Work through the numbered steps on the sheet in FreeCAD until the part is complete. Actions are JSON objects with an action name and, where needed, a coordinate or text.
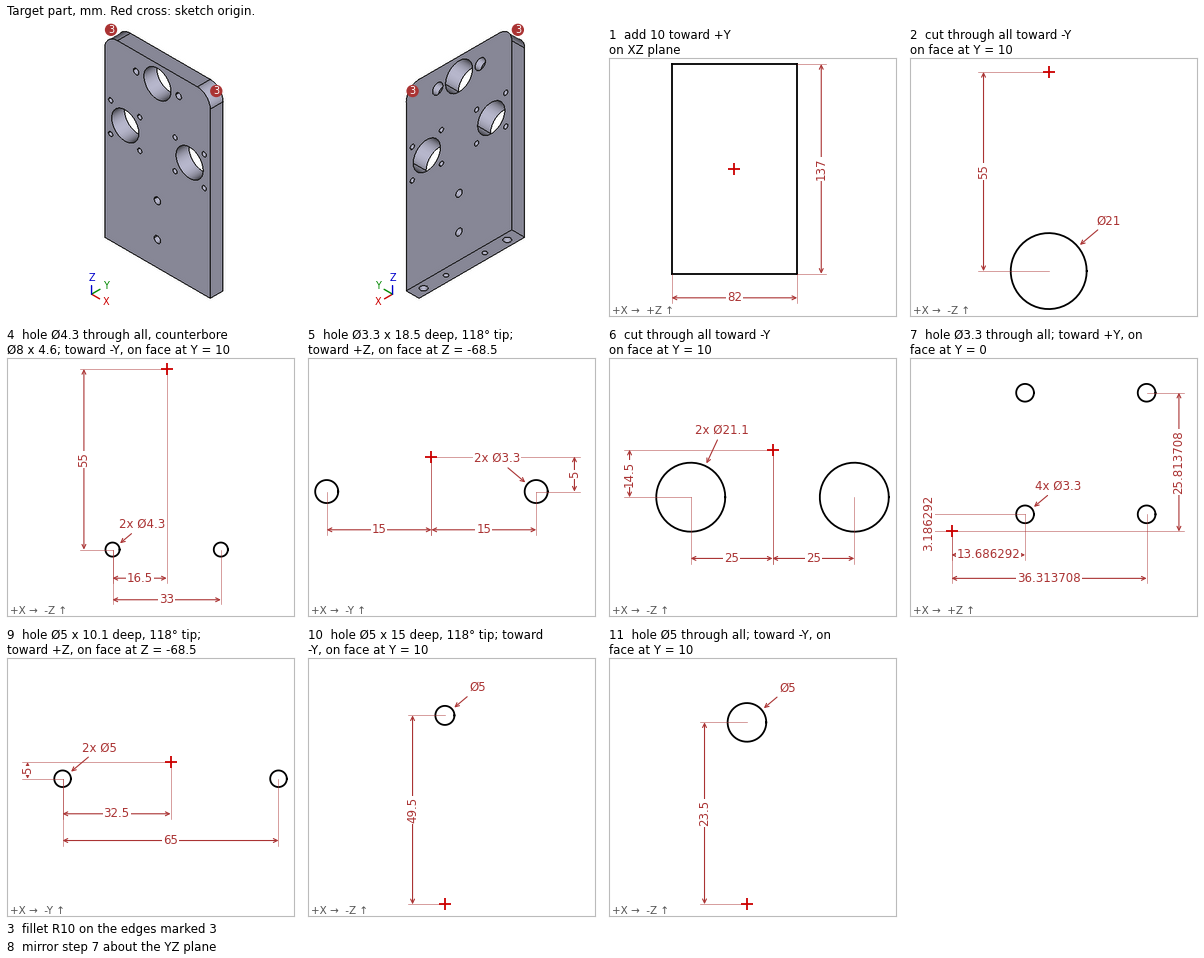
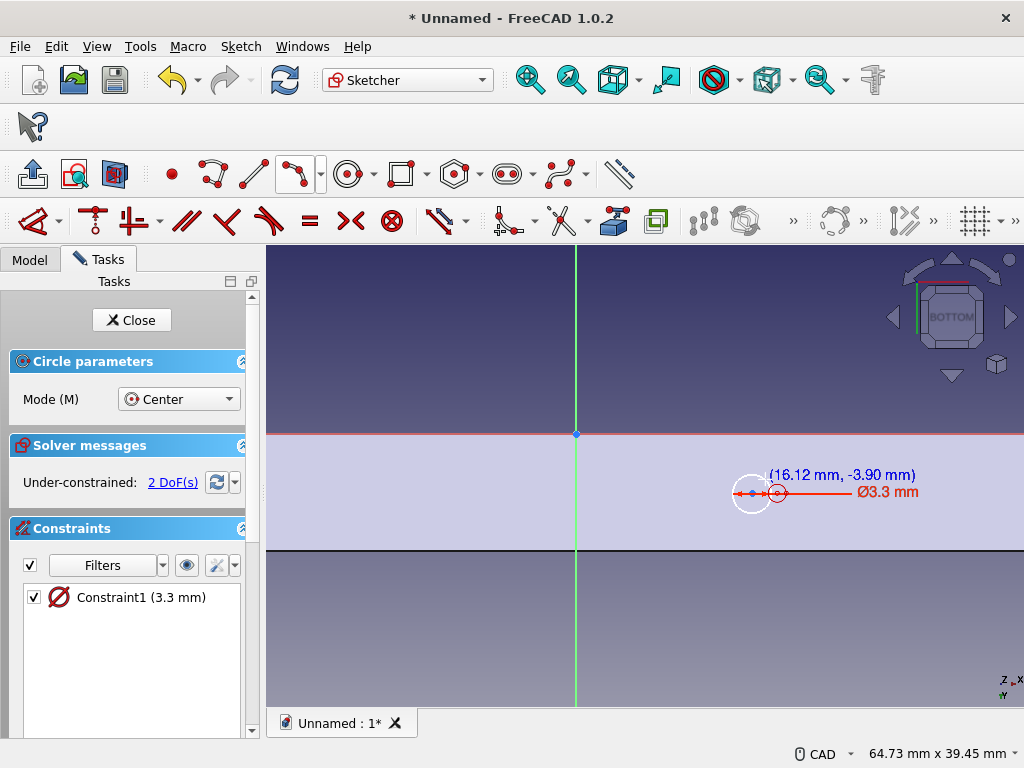
{"action": "left_click", "coordinate": [401, 493]}
{"action": "mouse_move", "coordinate": [414, 479]}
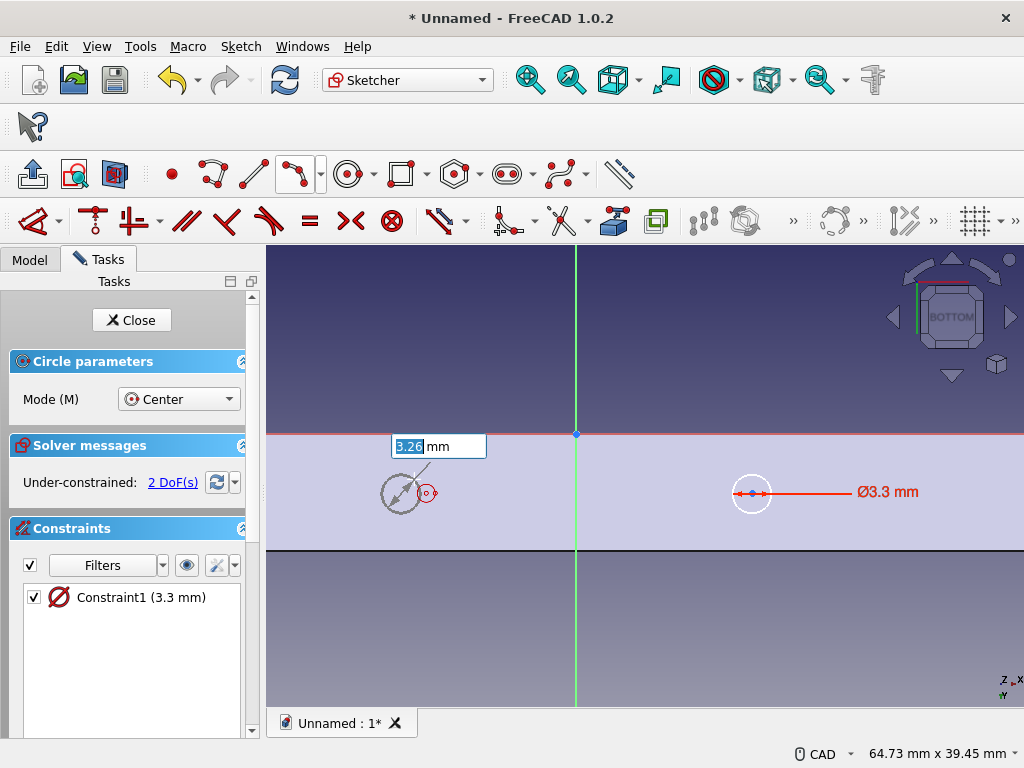
{"action": "type", "text": "3.3"}
{"action": "key", "text": "Return"}
{"action": "key", "text": "Escape"}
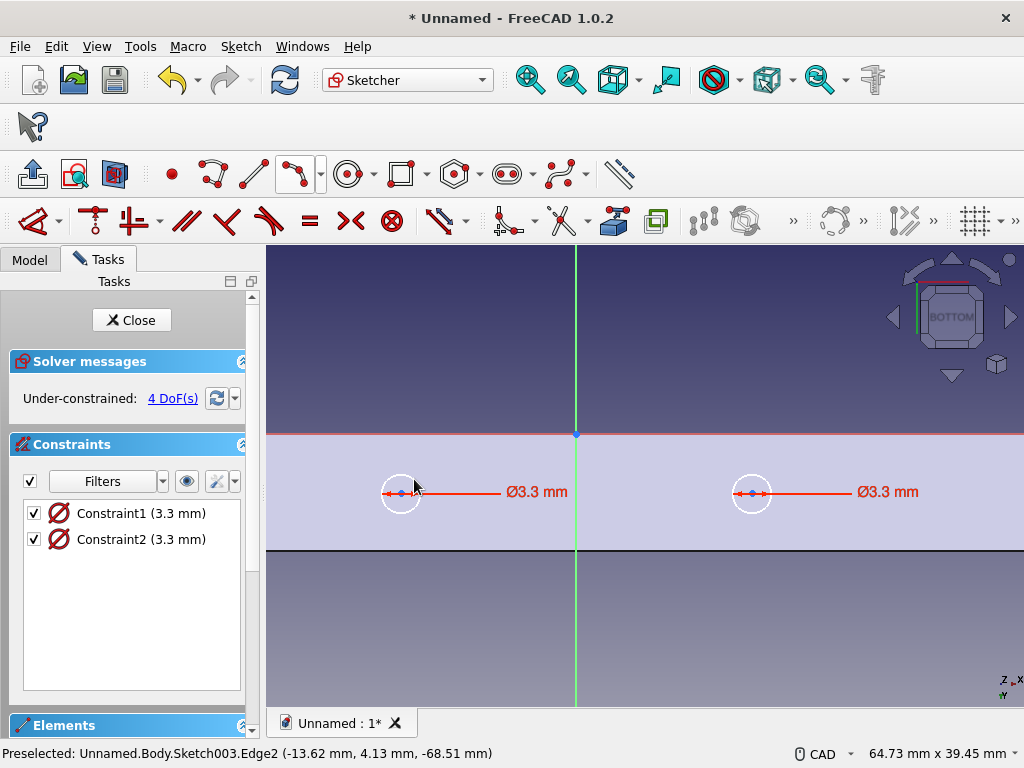
{"action": "left_click", "coordinate": [752, 494]}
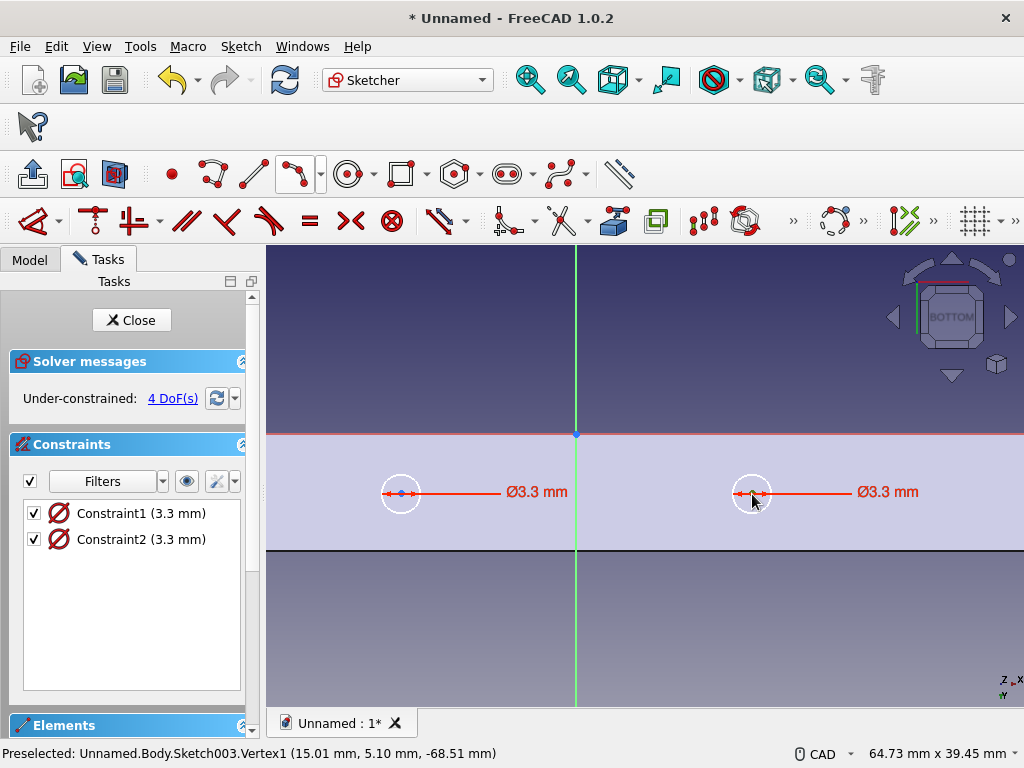
{"action": "left_click", "coordinate": [401, 494]}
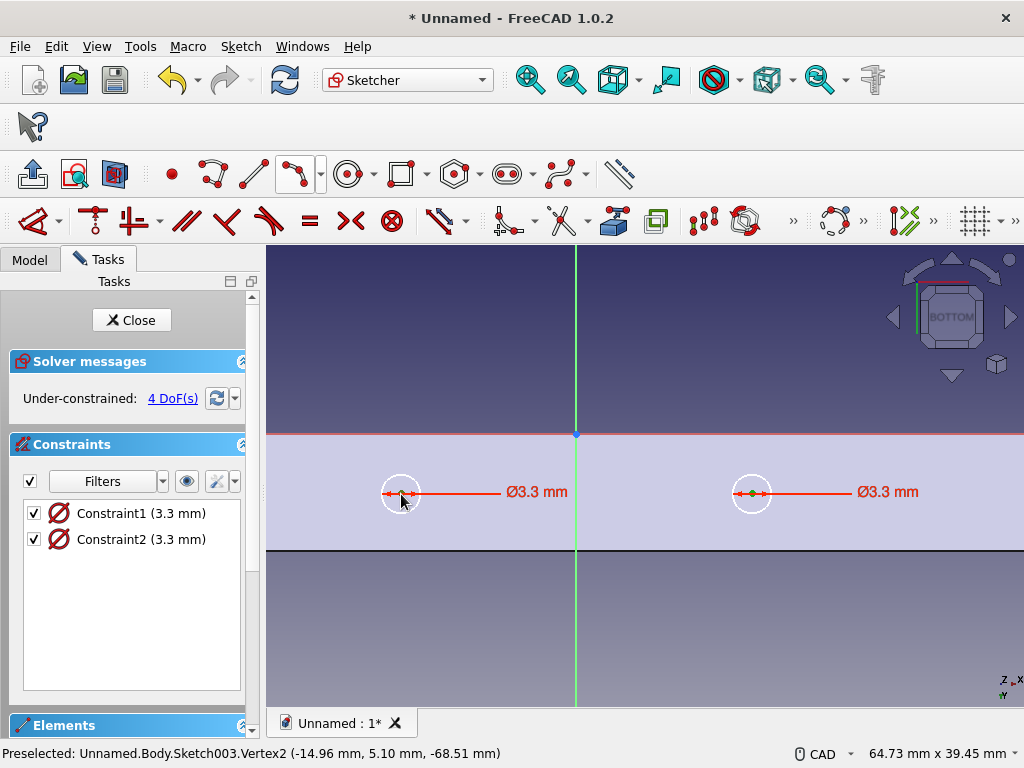
{"action": "left_click", "coordinate": [160, 222]}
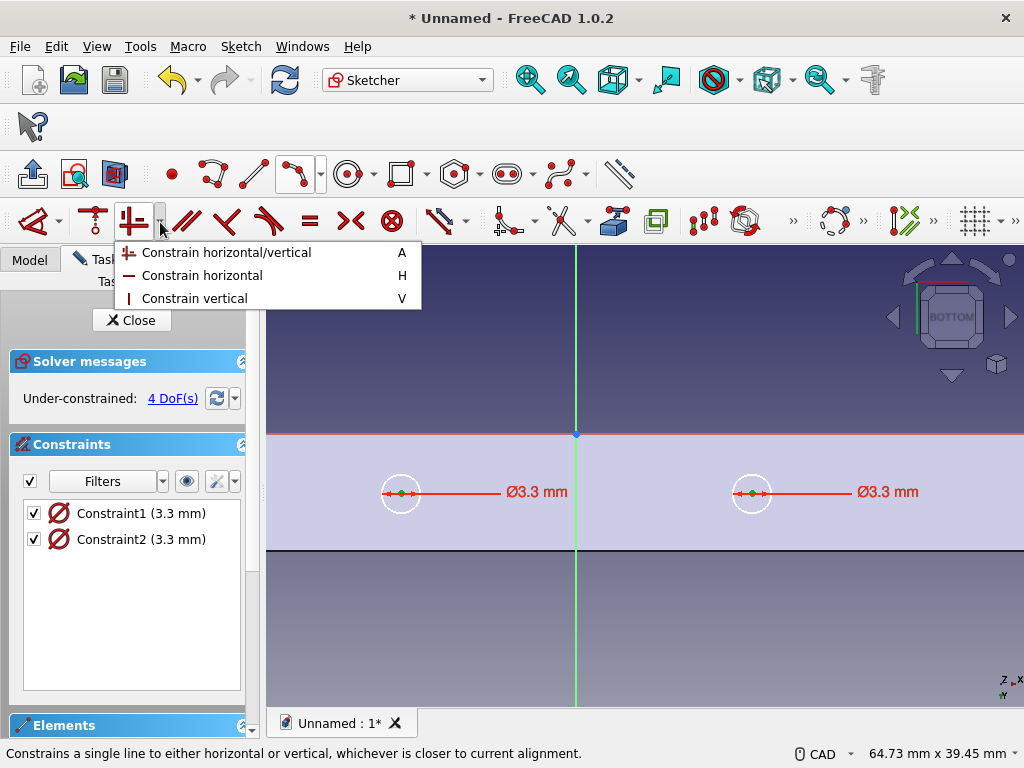
{"action": "left_click", "coordinate": [268, 276]}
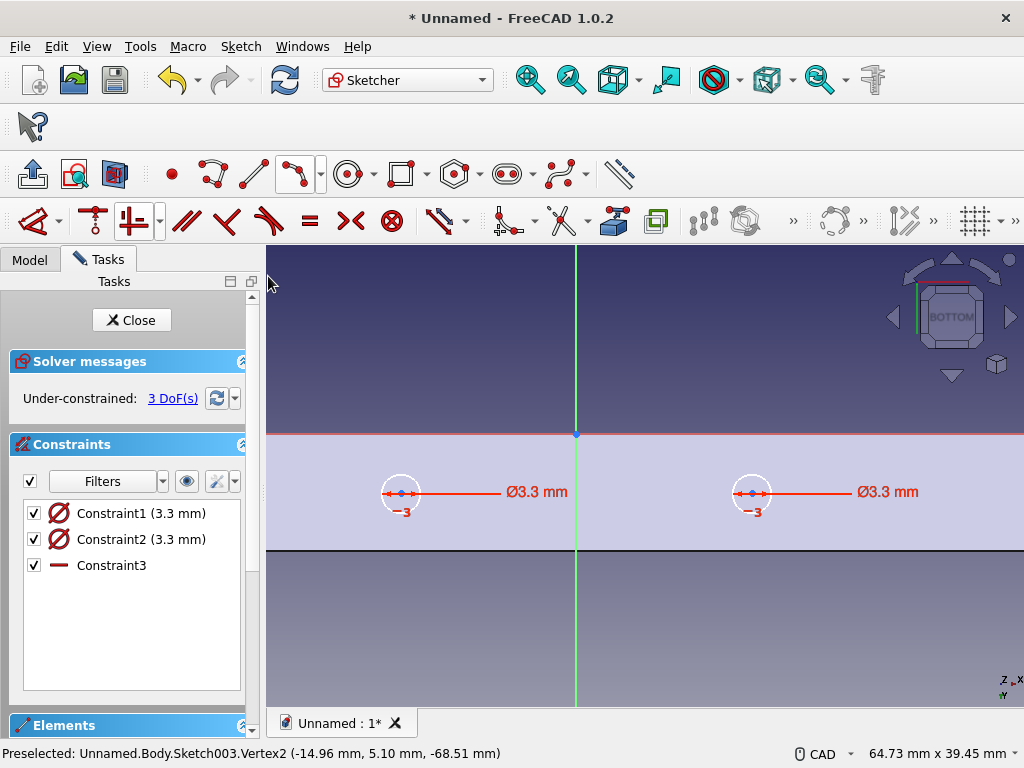
{"action": "left_click", "coordinate": [32, 222]}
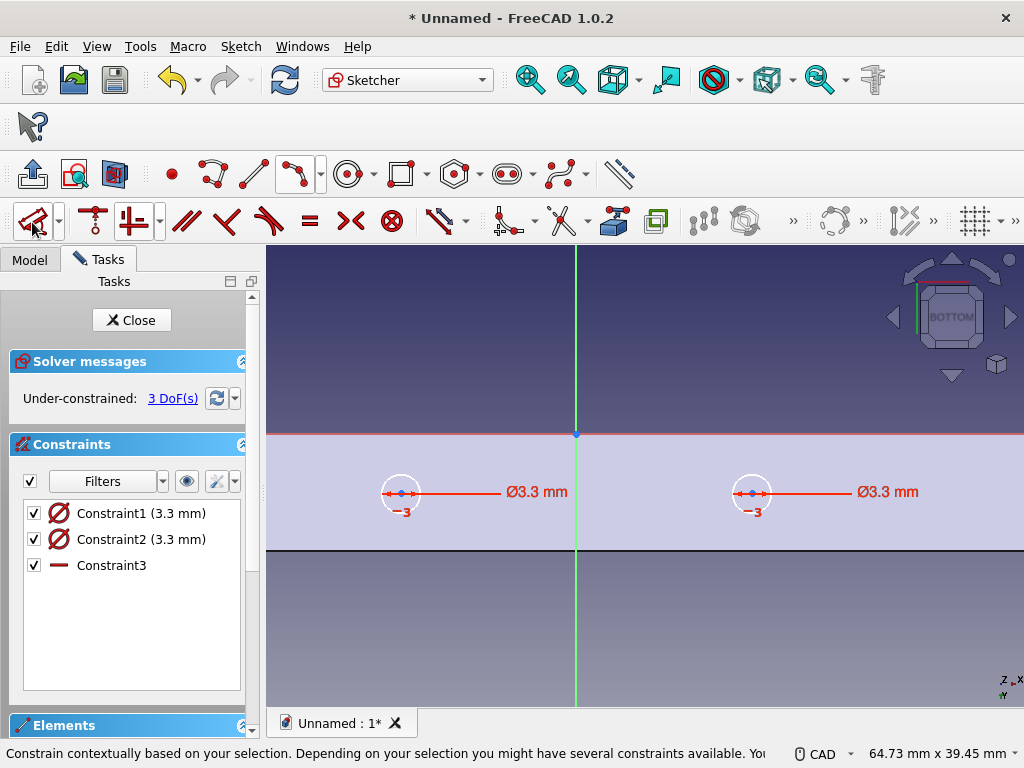
{"action": "left_click", "coordinate": [752, 494]}
{"action": "left_click", "coordinate": [786, 464]}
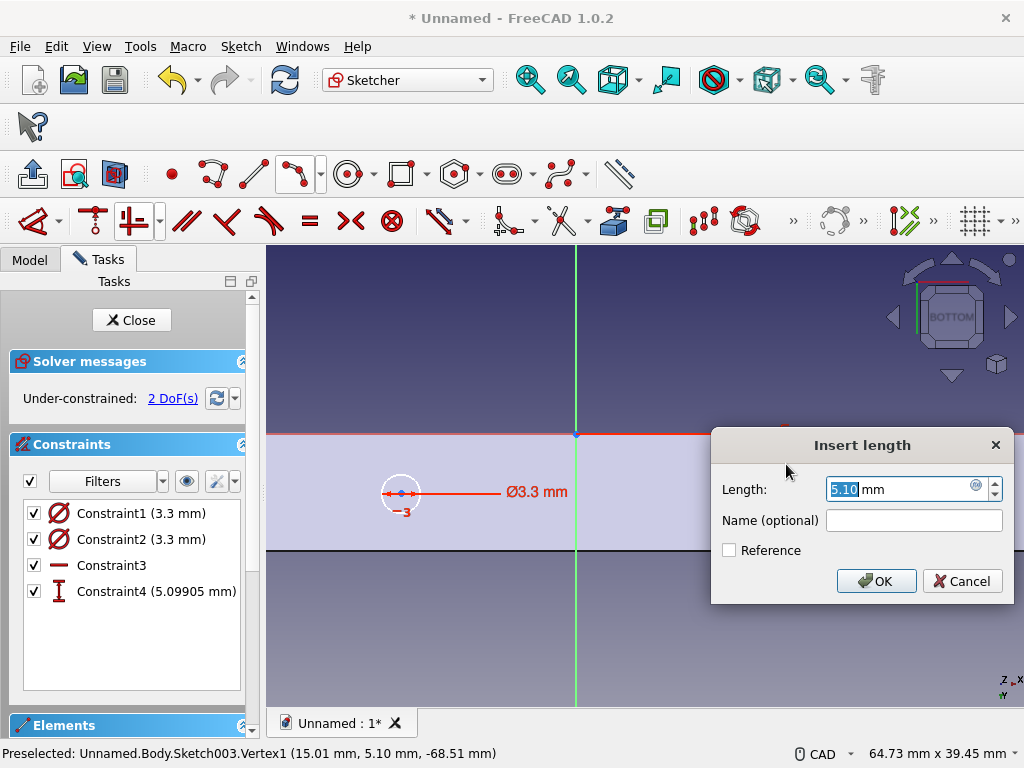
{"action": "type", "text": "5"}
{"action": "key", "text": "Return"}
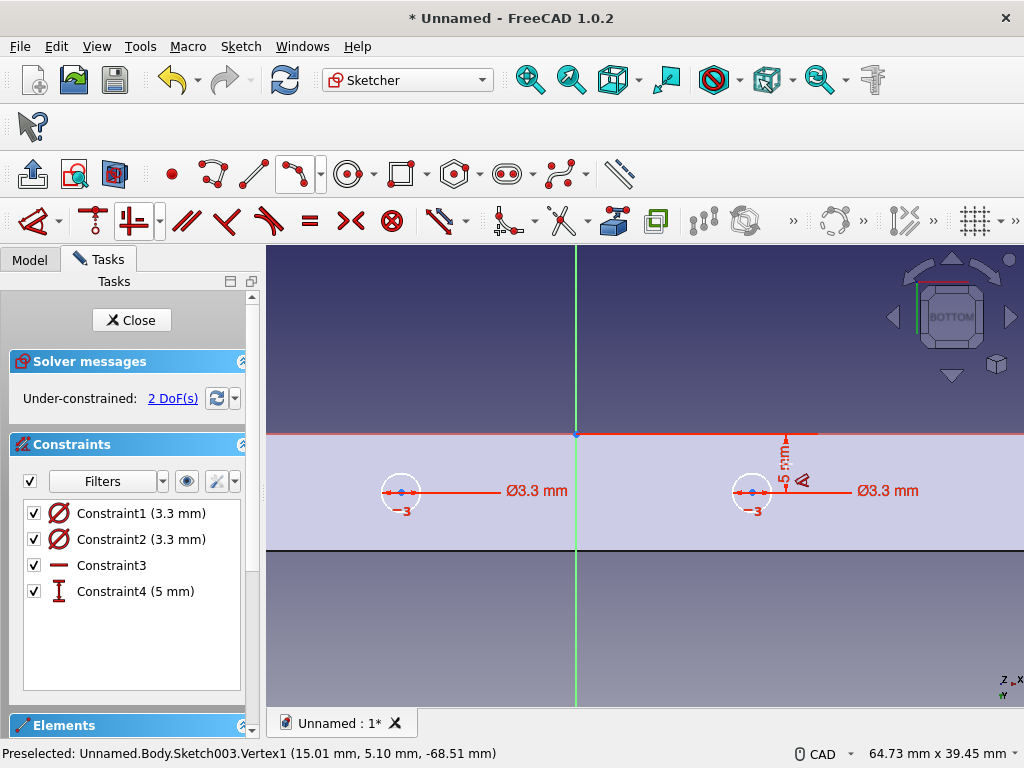
{"action": "left_click", "coordinate": [752, 493]}
{"action": "left_click", "coordinate": [664, 400]}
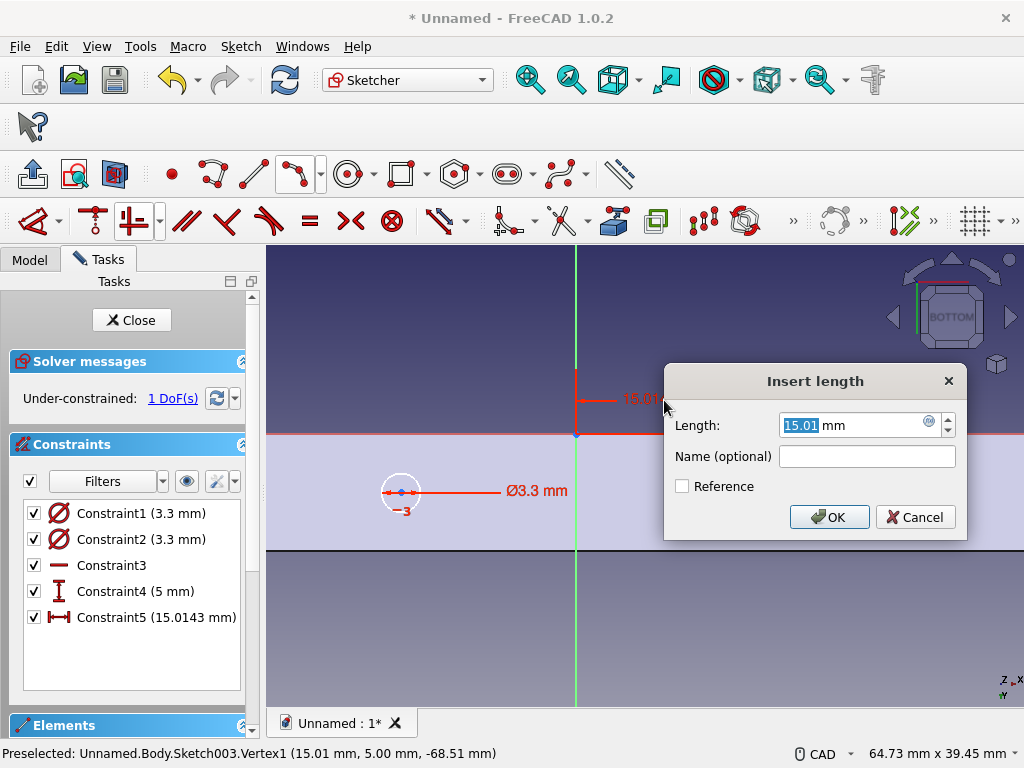
{"action": "type", "text": "15"}
{"action": "key", "text": "Return"}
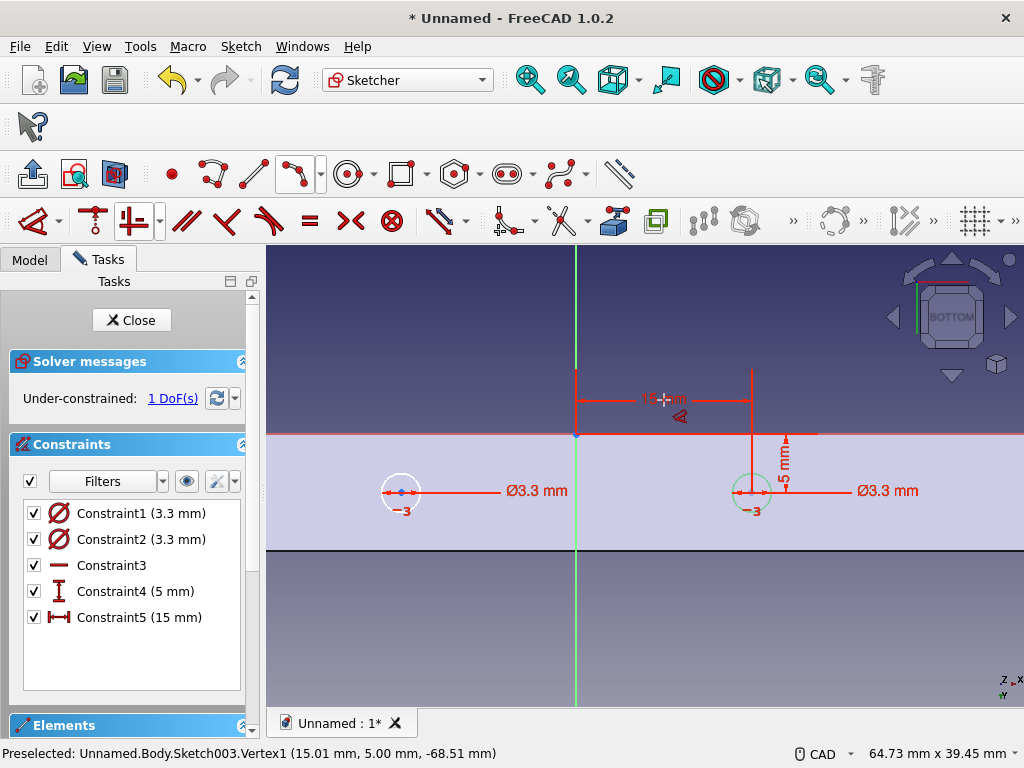
{"action": "left_click", "coordinate": [401, 493]}
{"action": "left_click", "coordinate": [489, 400]}